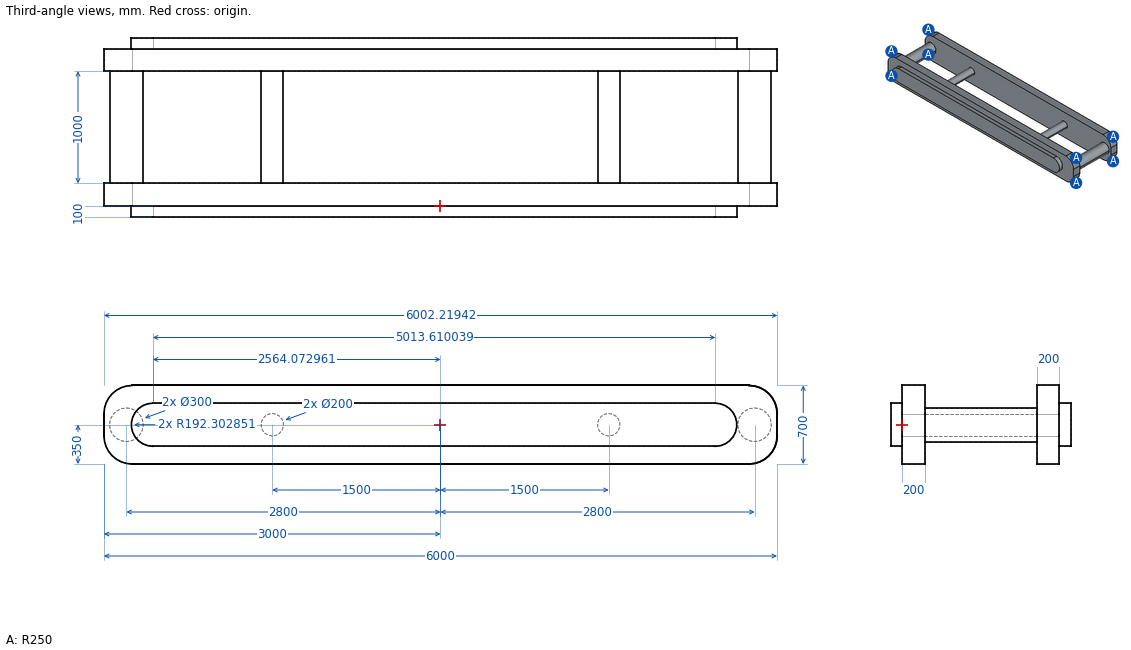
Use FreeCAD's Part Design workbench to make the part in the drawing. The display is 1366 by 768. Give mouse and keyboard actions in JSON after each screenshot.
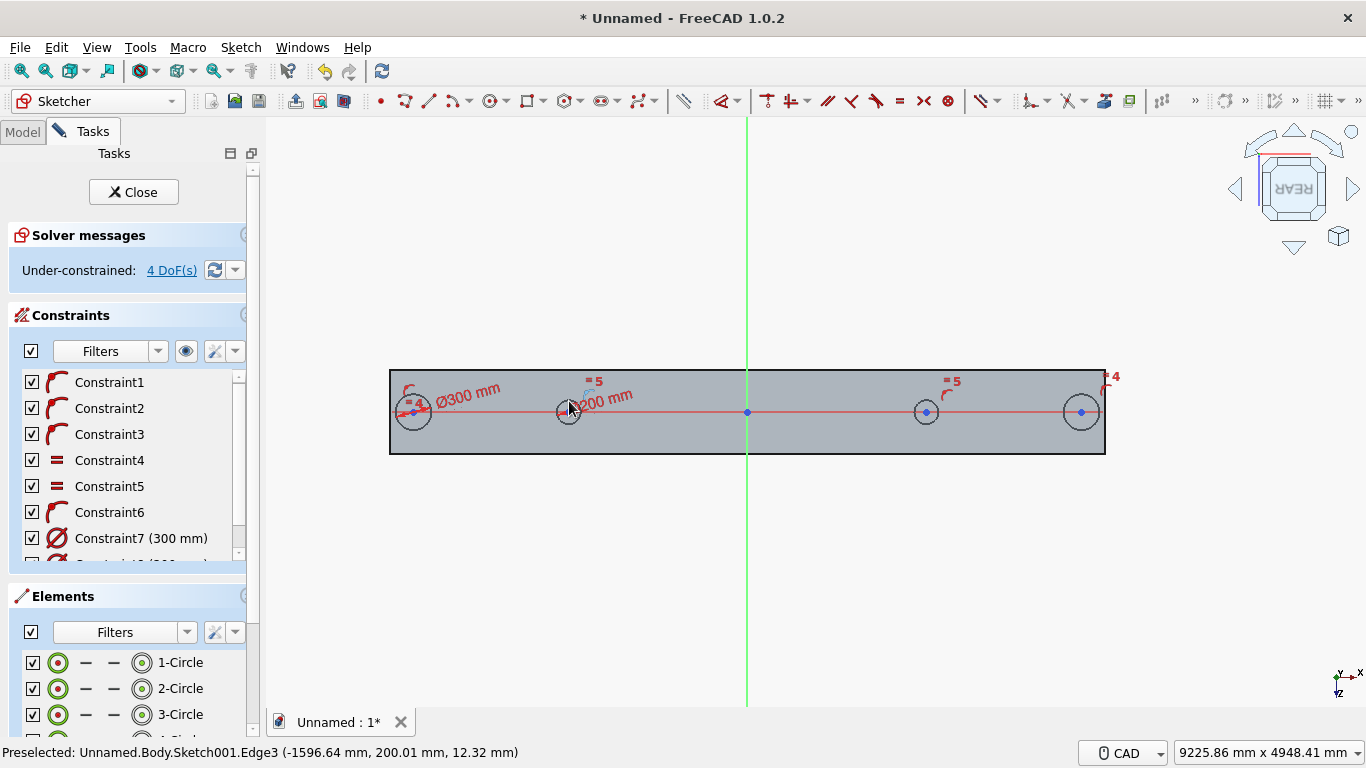
{"action": "left_click", "coordinate": [413, 412]}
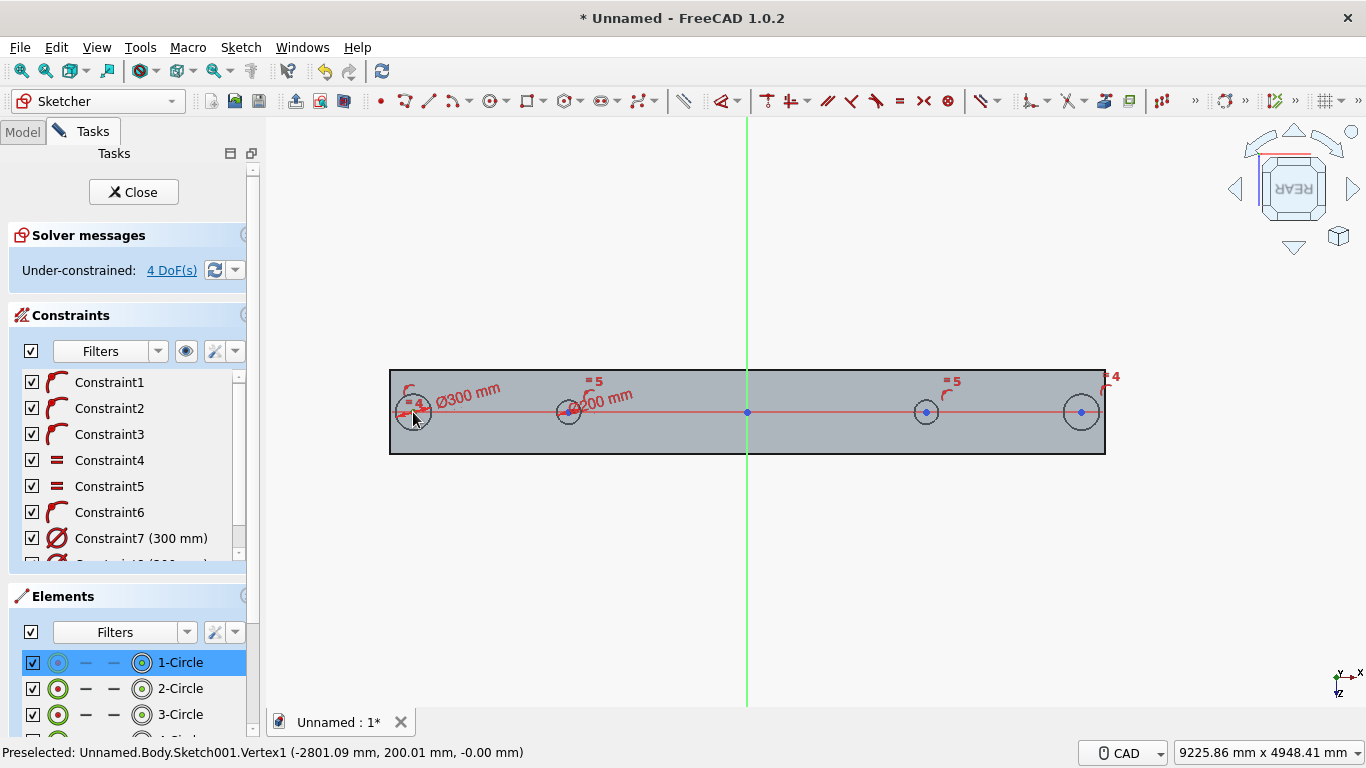
{"action": "left_click", "coordinate": [740, 102]}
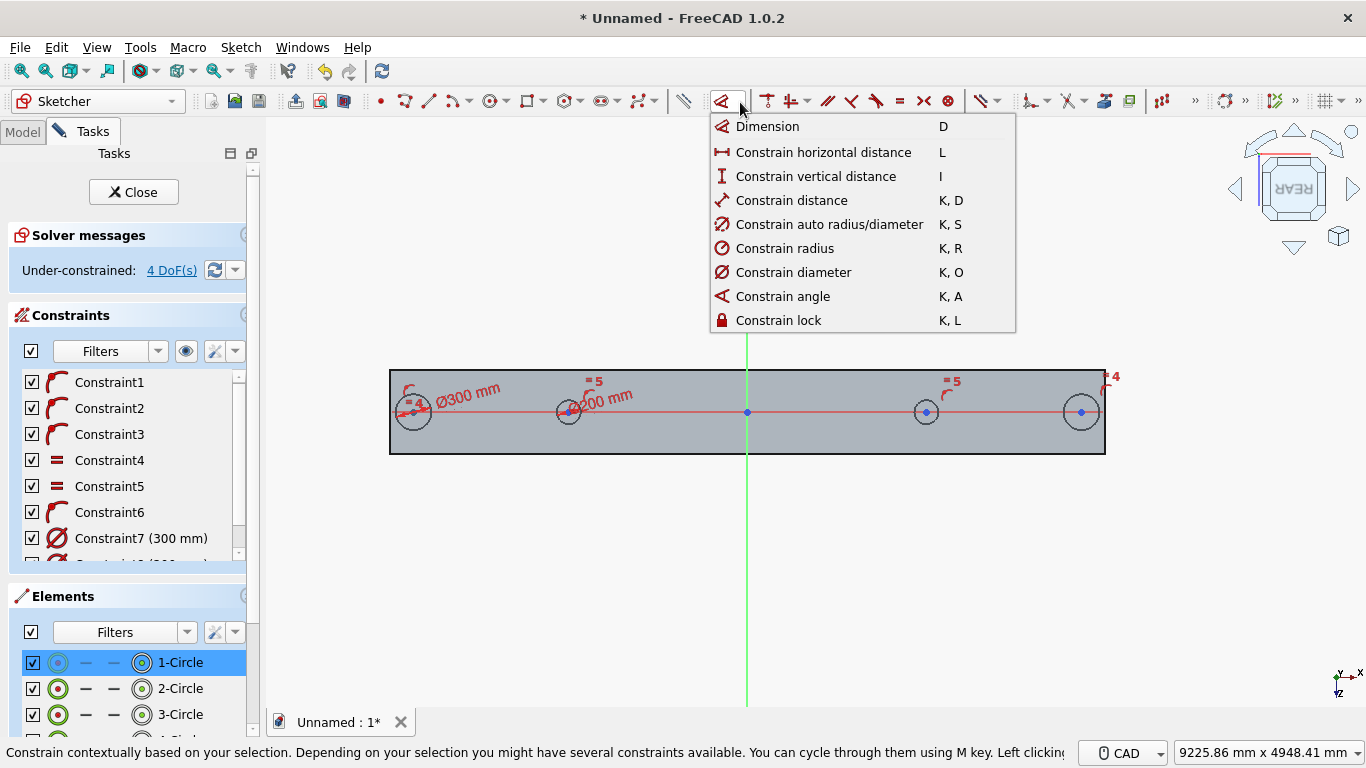
{"action": "left_click", "coordinate": [863, 152]}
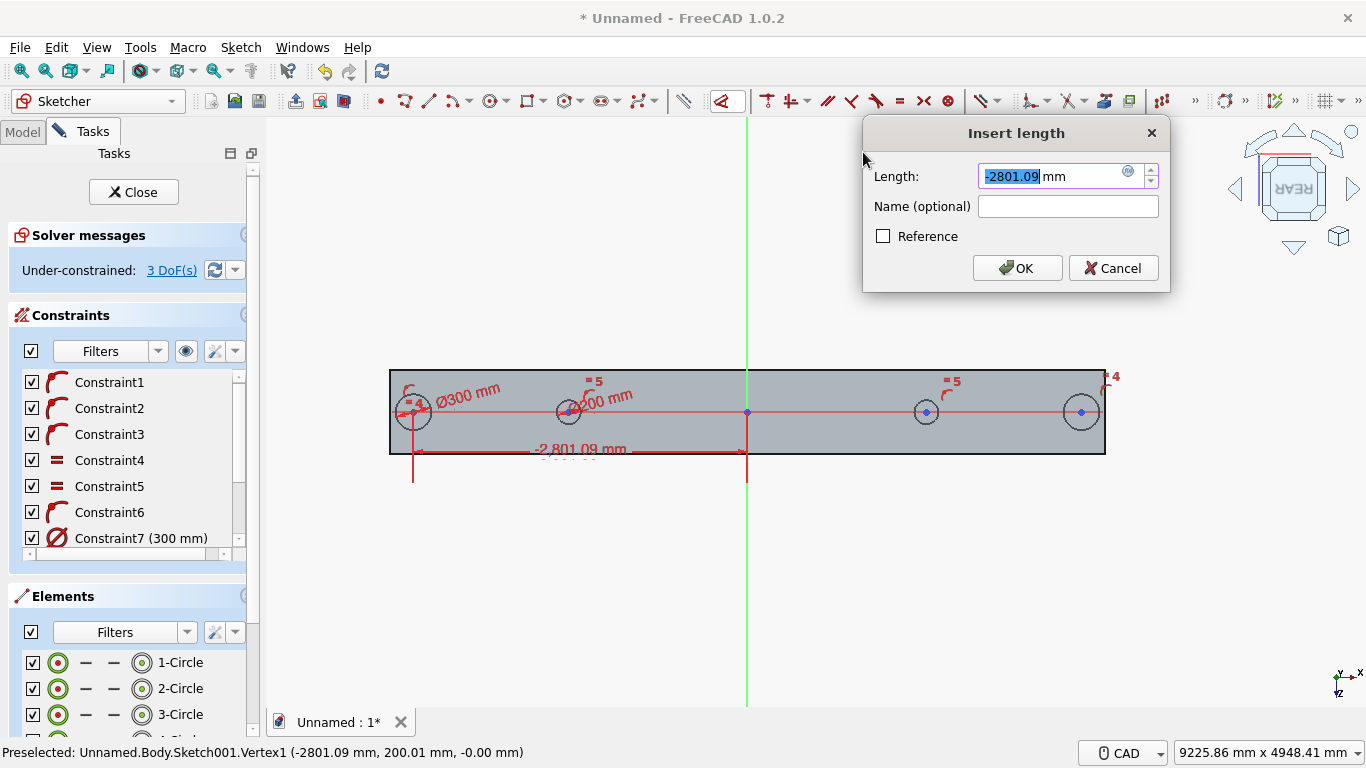
{"action": "type", "text": "-2800"}
{"action": "key", "text": "Return"}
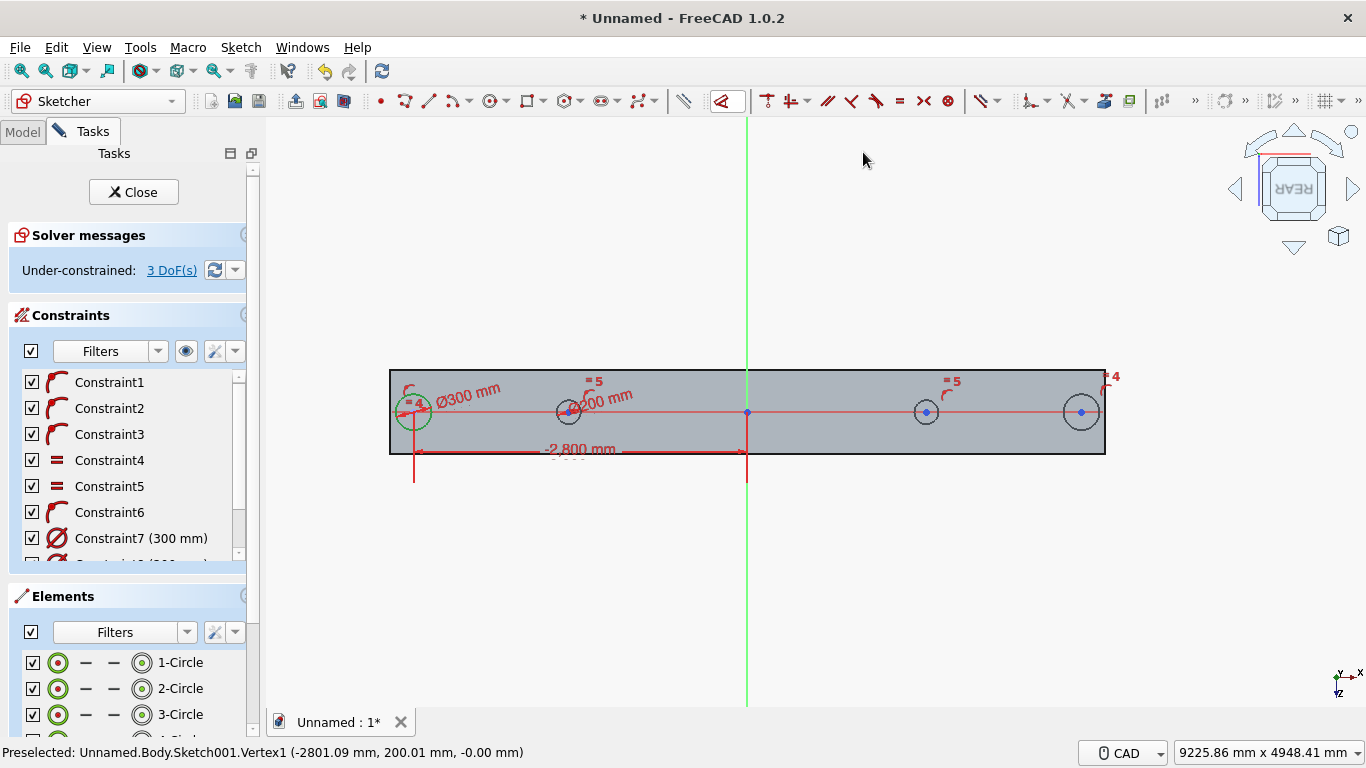
{"action": "left_click", "coordinate": [1082, 412]}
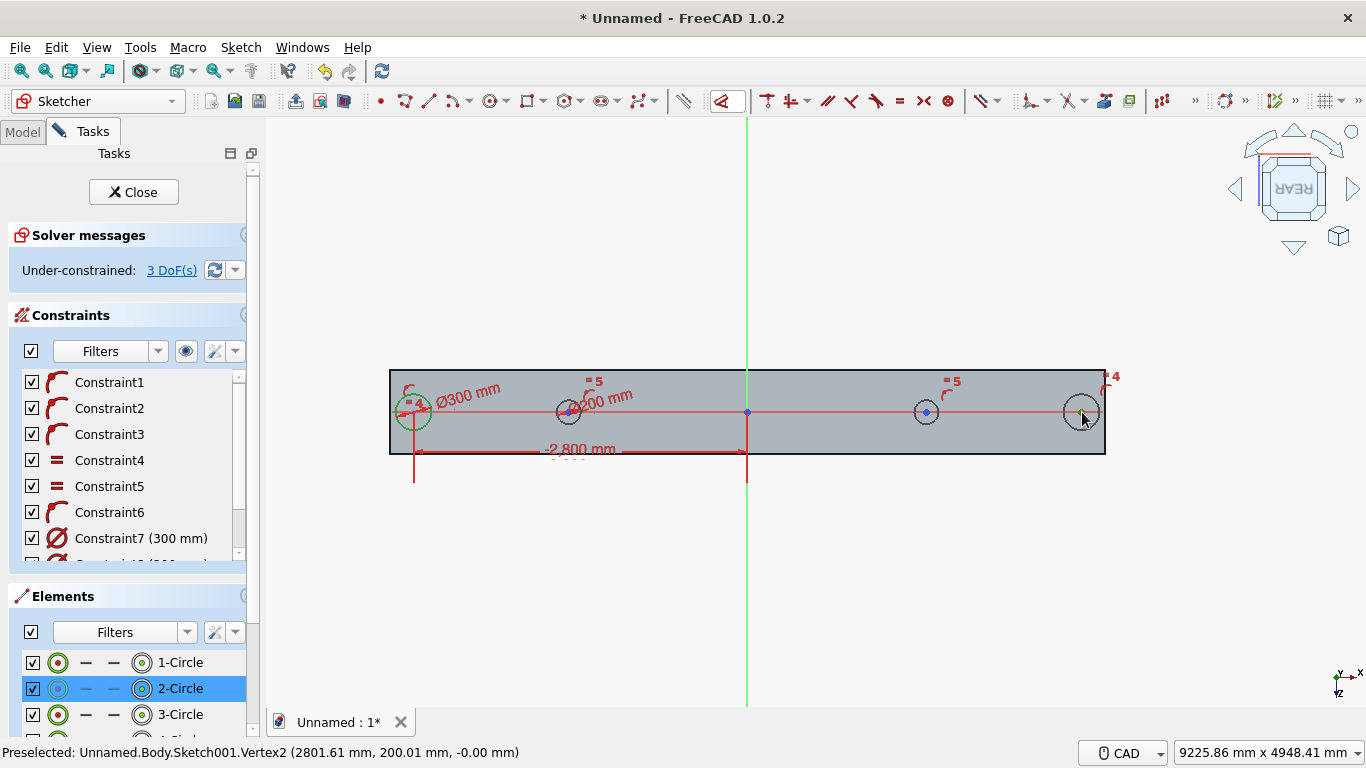
{"action": "left_click", "coordinate": [740, 102]}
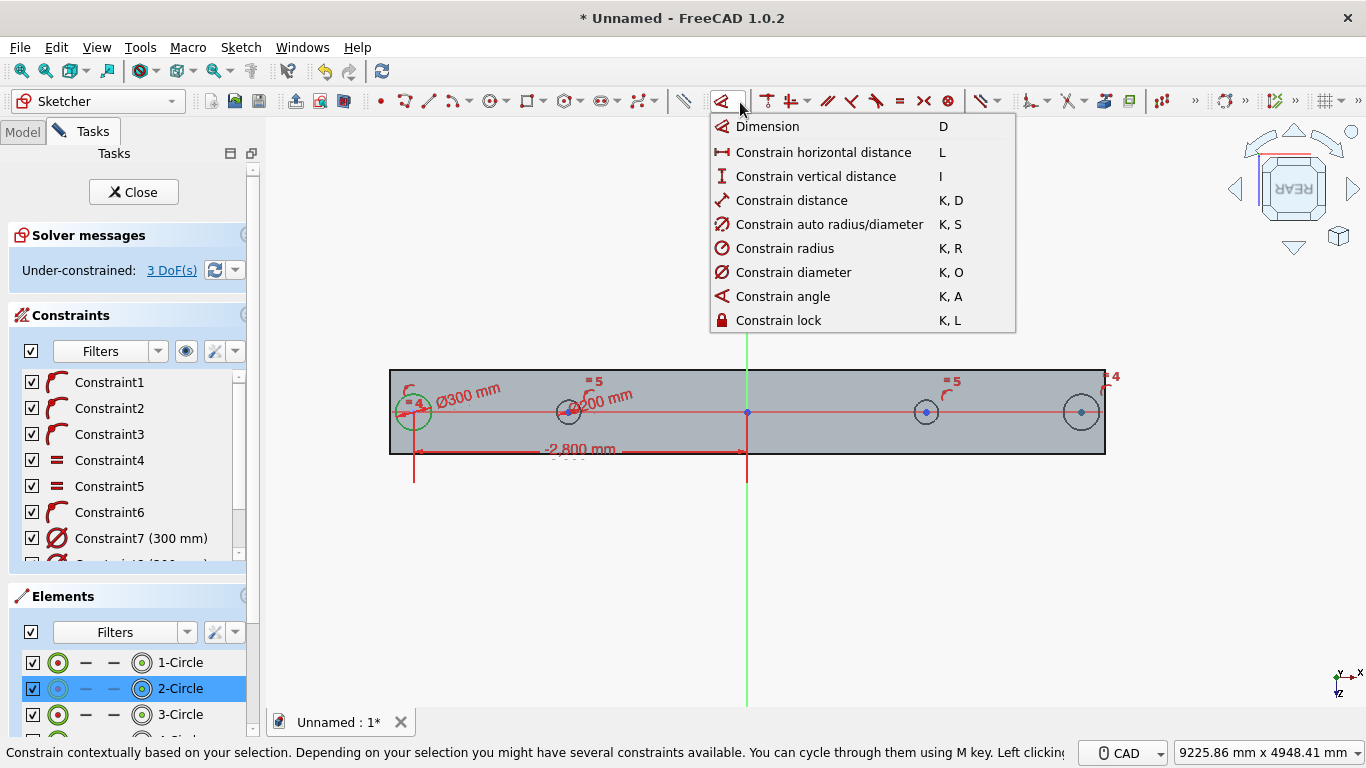
{"action": "left_click", "coordinate": [863, 152]}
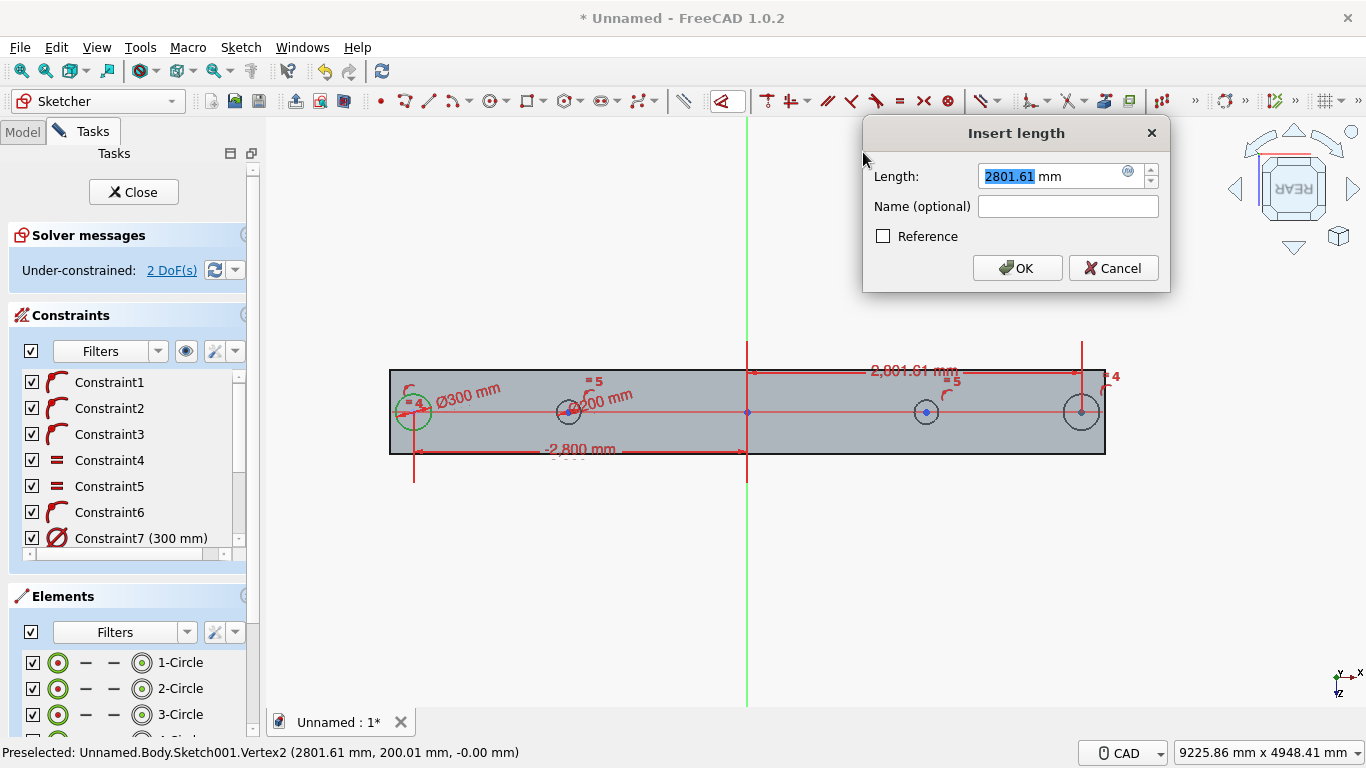
{"action": "type", "text": "2800"}
{"action": "key", "text": "Return"}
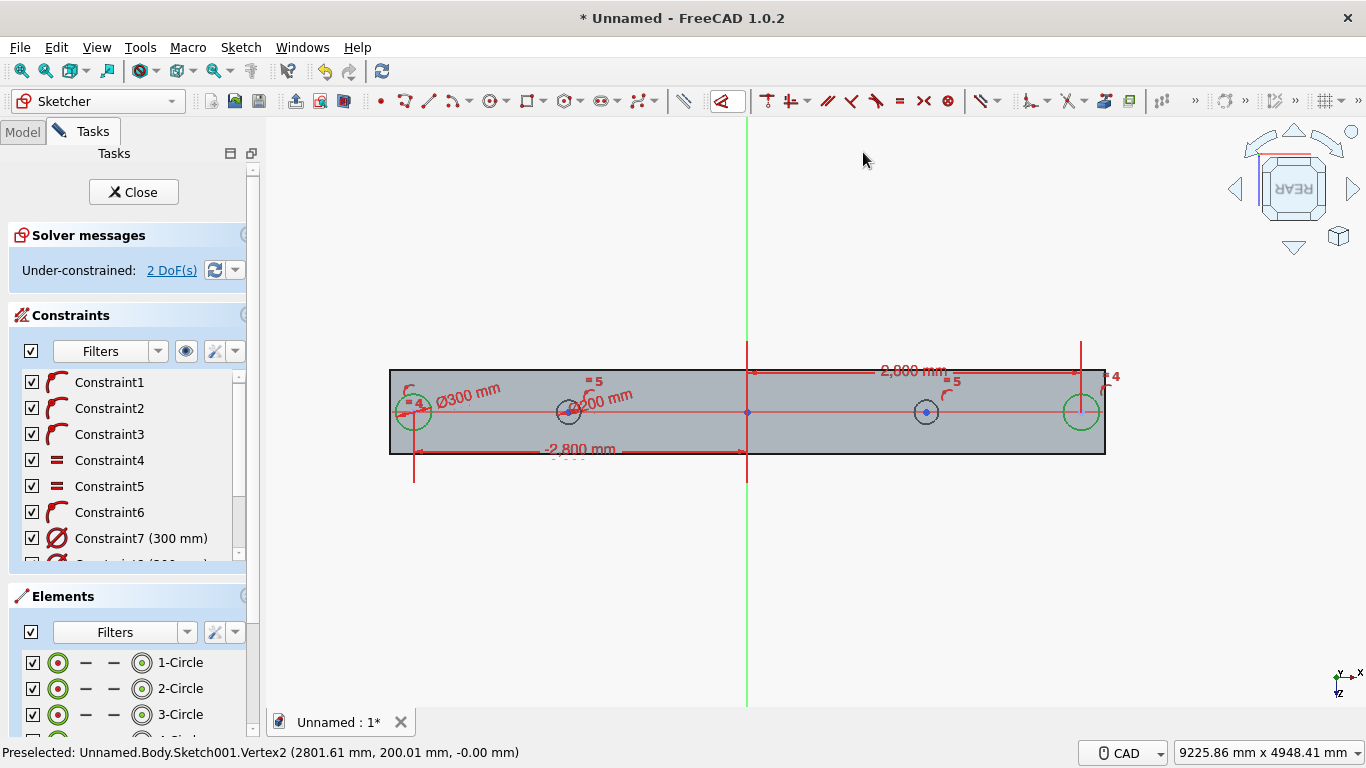
{"action": "left_click", "coordinate": [569, 412]}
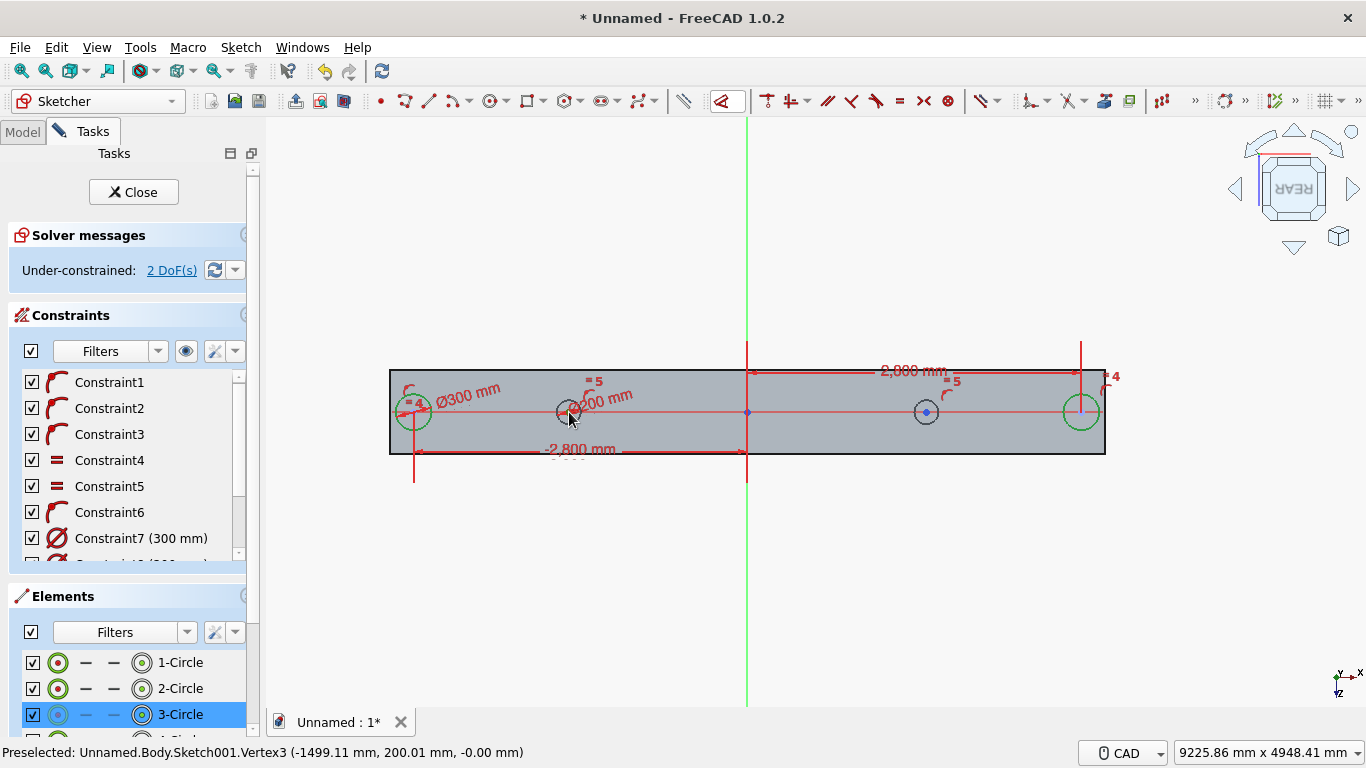
{"action": "key", "text": "l"}